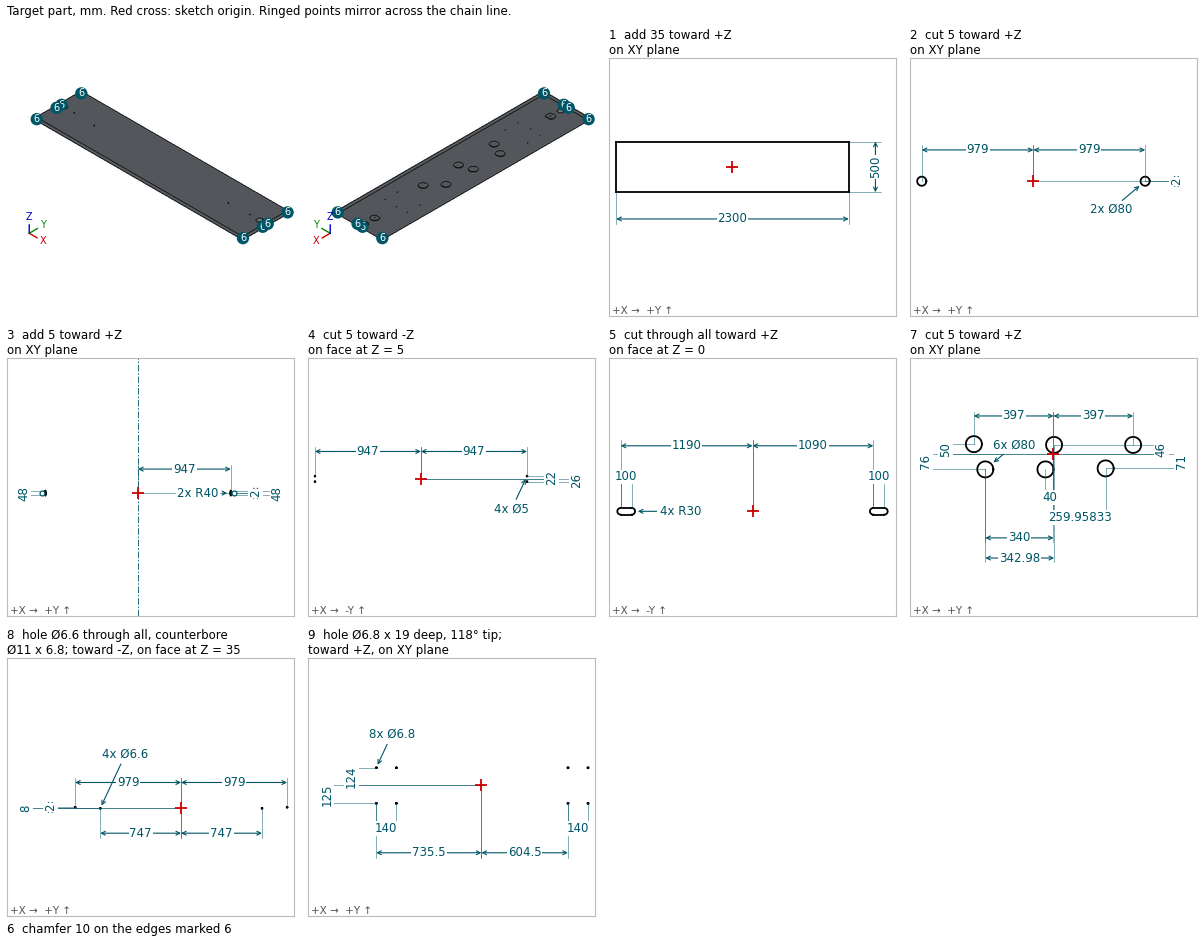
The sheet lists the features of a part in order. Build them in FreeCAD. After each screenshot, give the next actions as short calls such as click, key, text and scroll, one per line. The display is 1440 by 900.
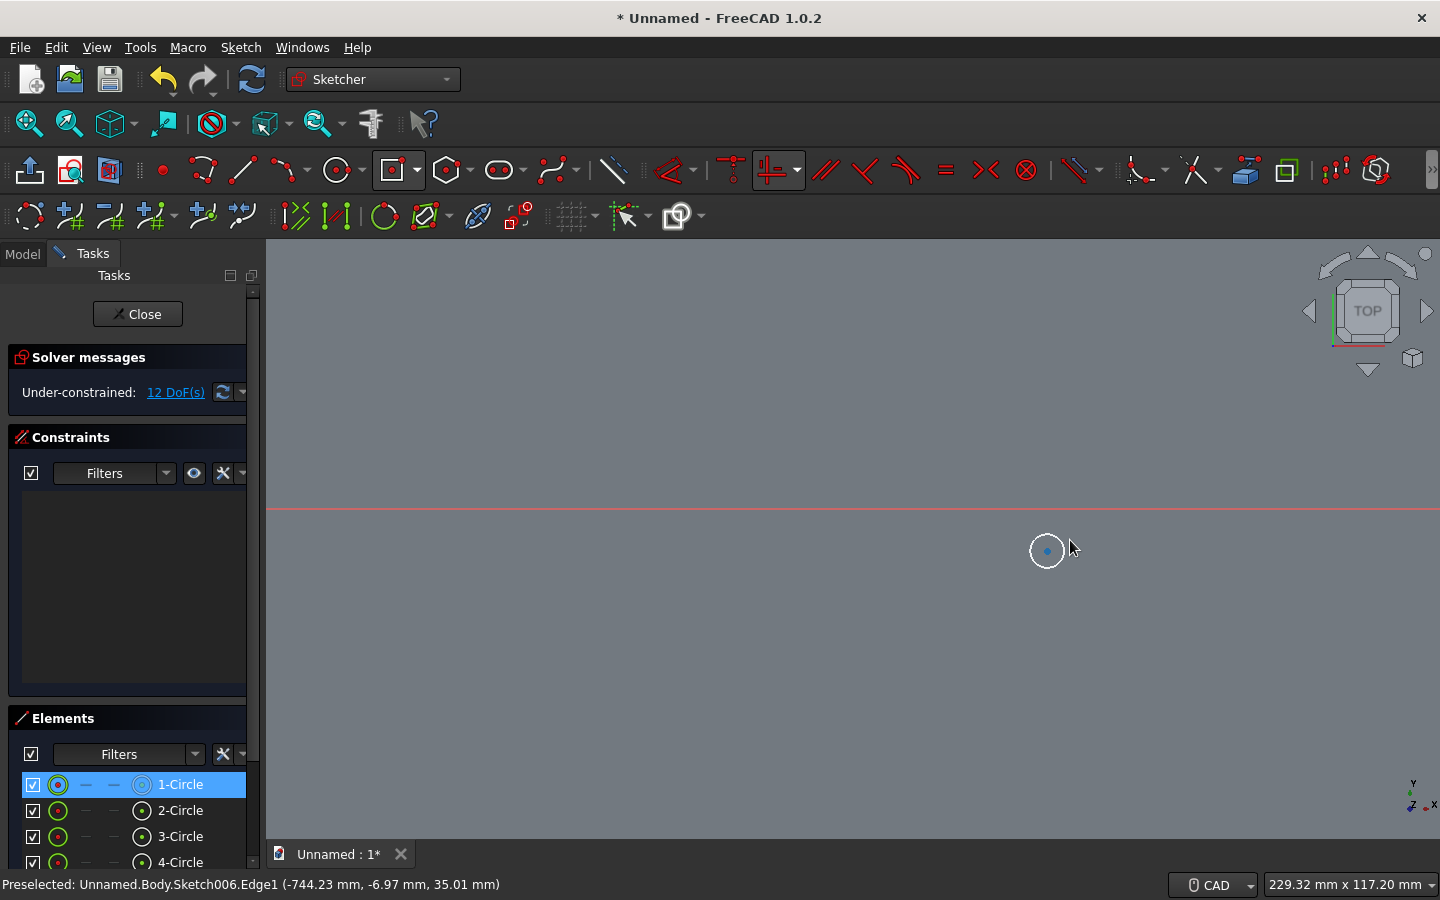
click(1059, 539)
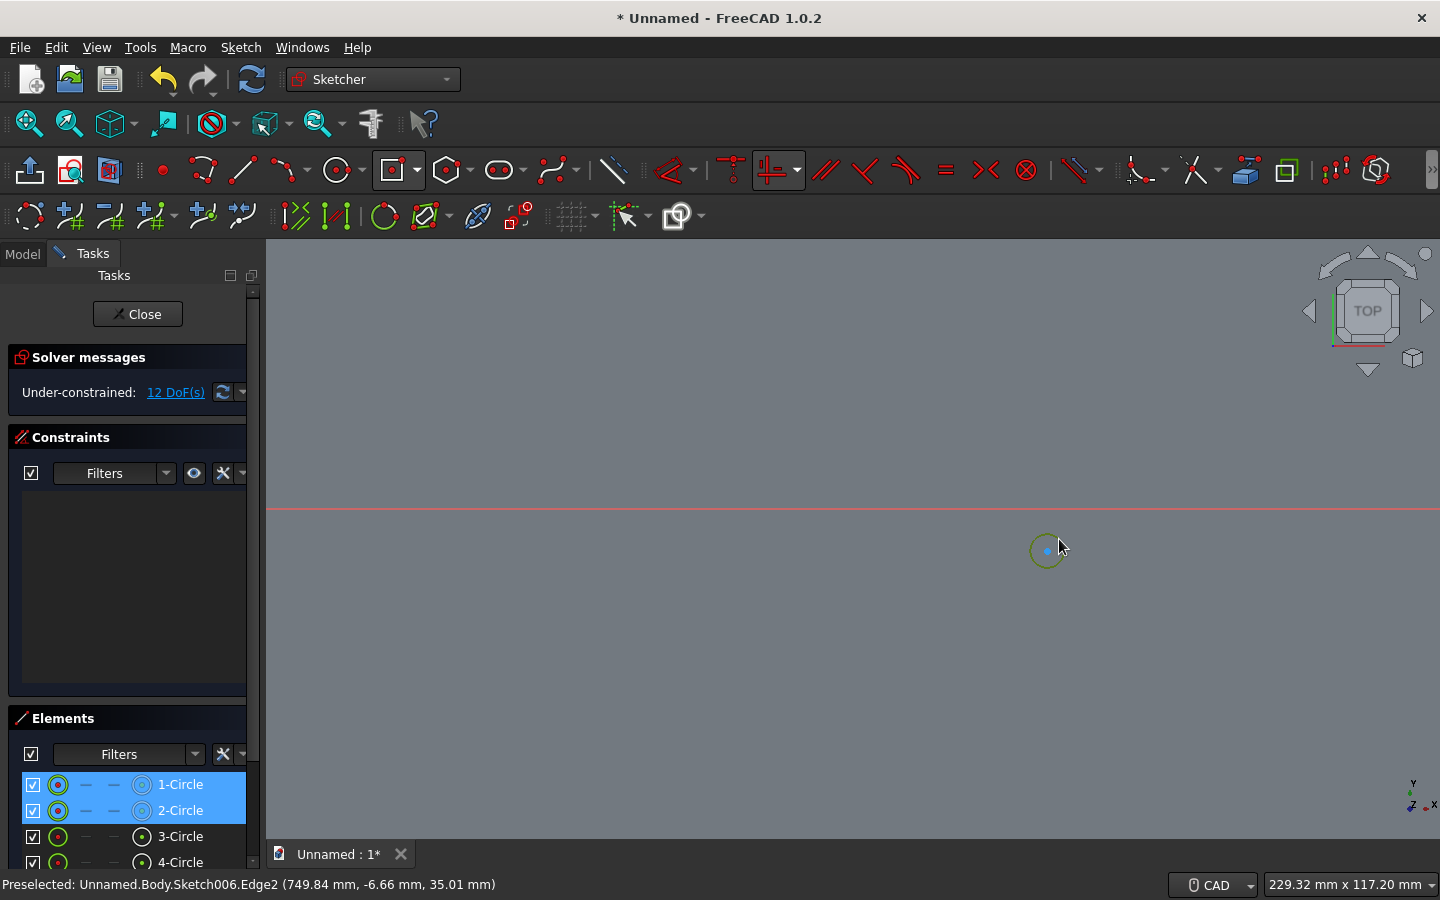
scroll(1070, 540, down, 13)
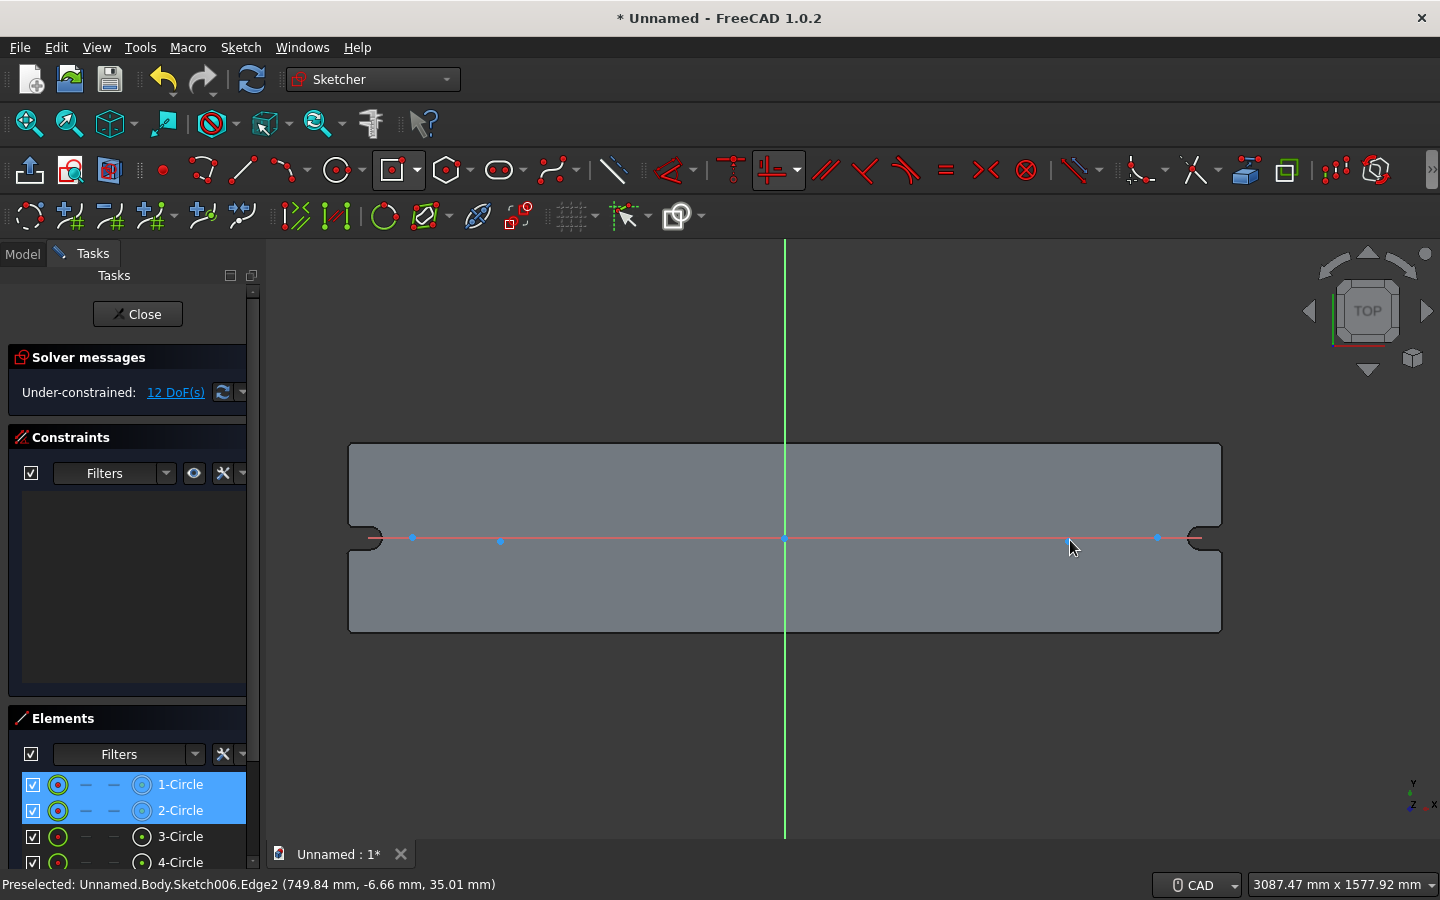
scroll(414, 537, up, 12)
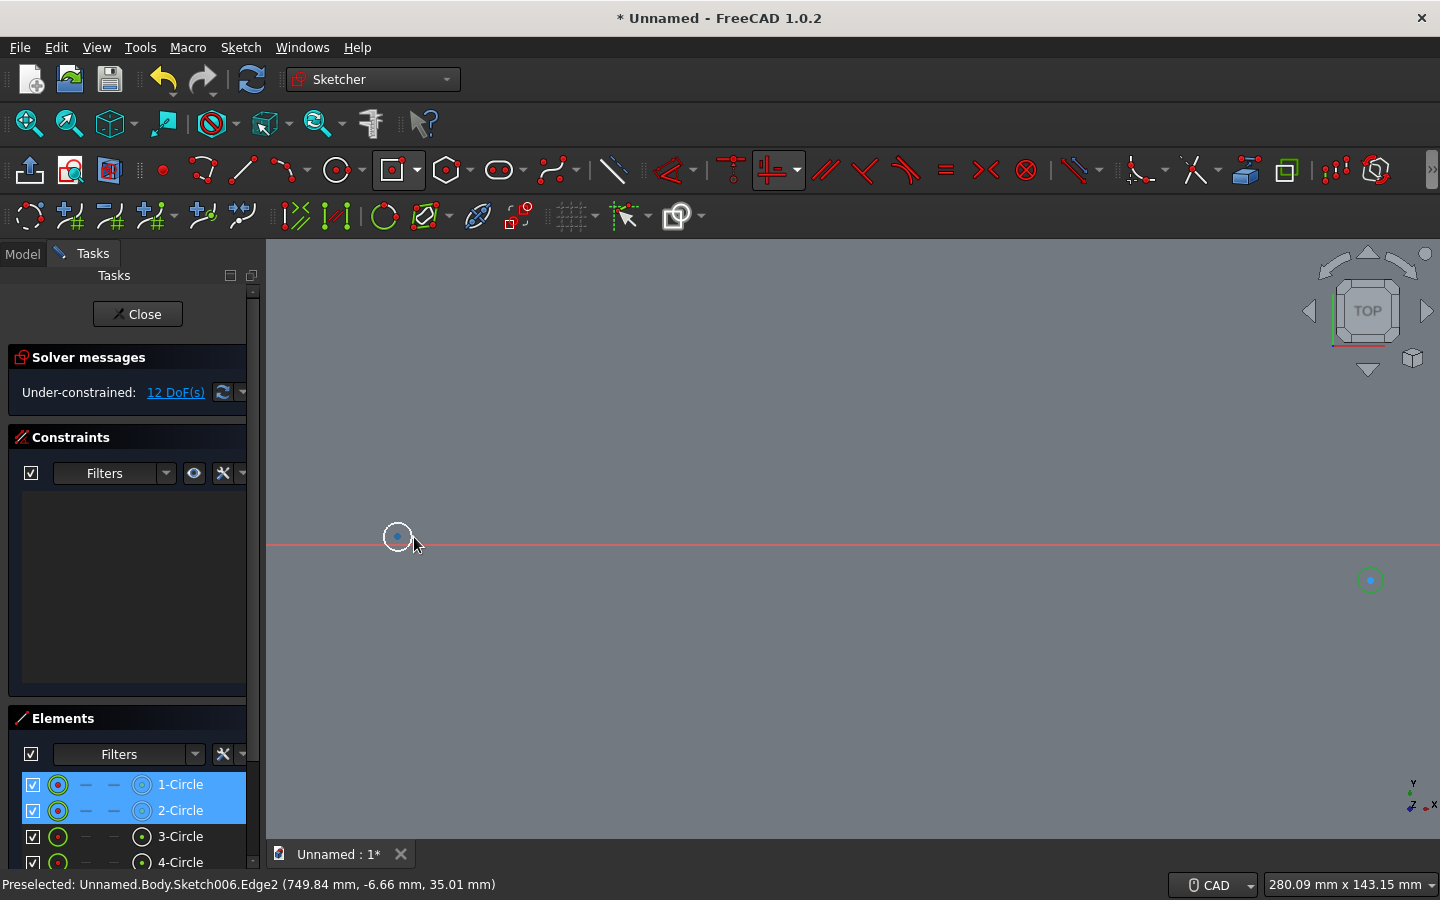
click(408, 527)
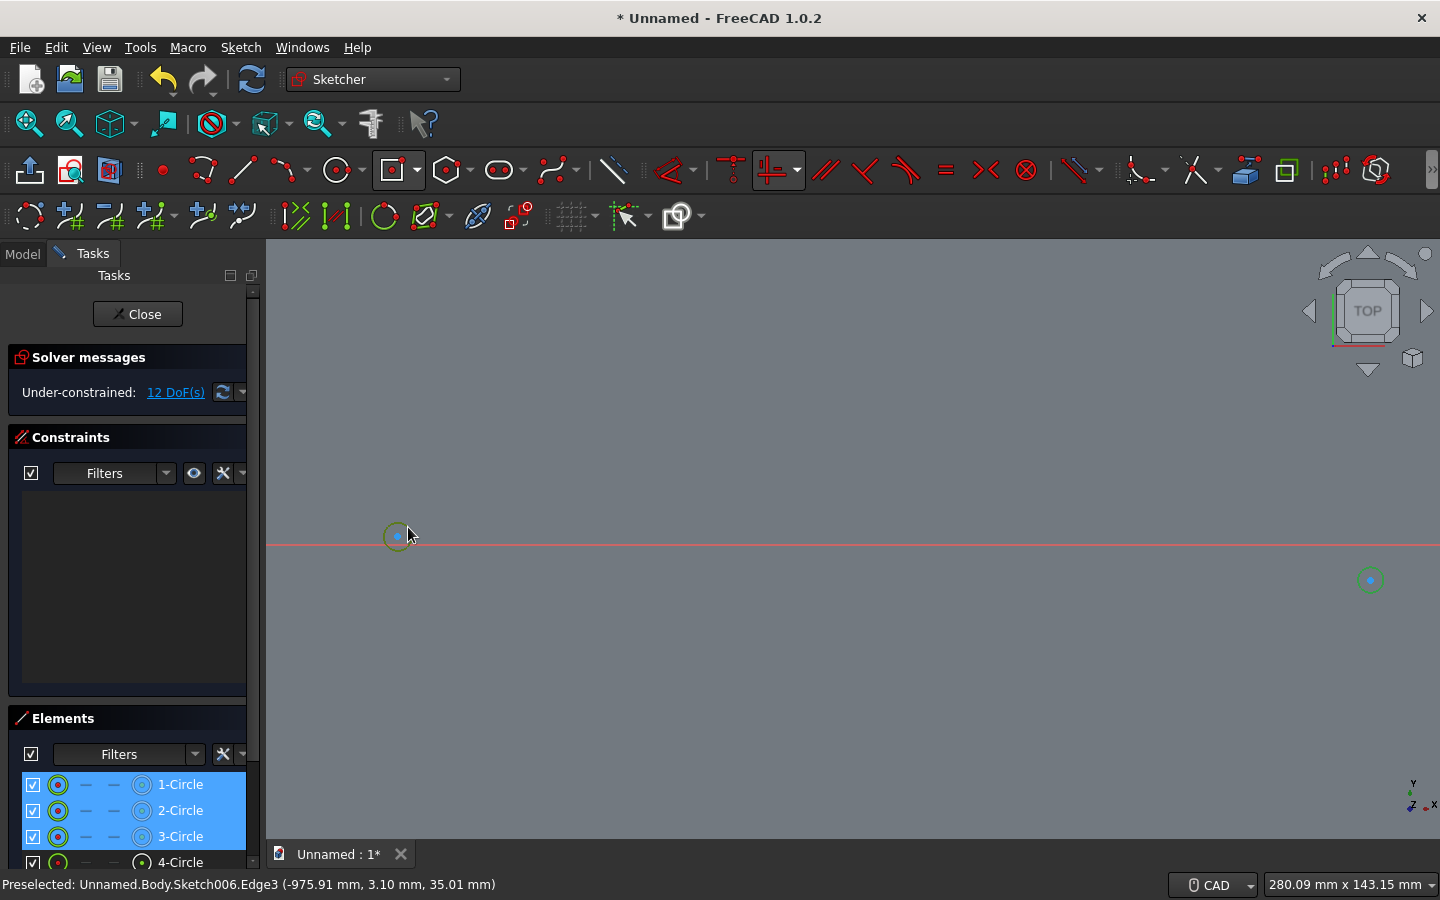
scroll(414, 537, down, 12)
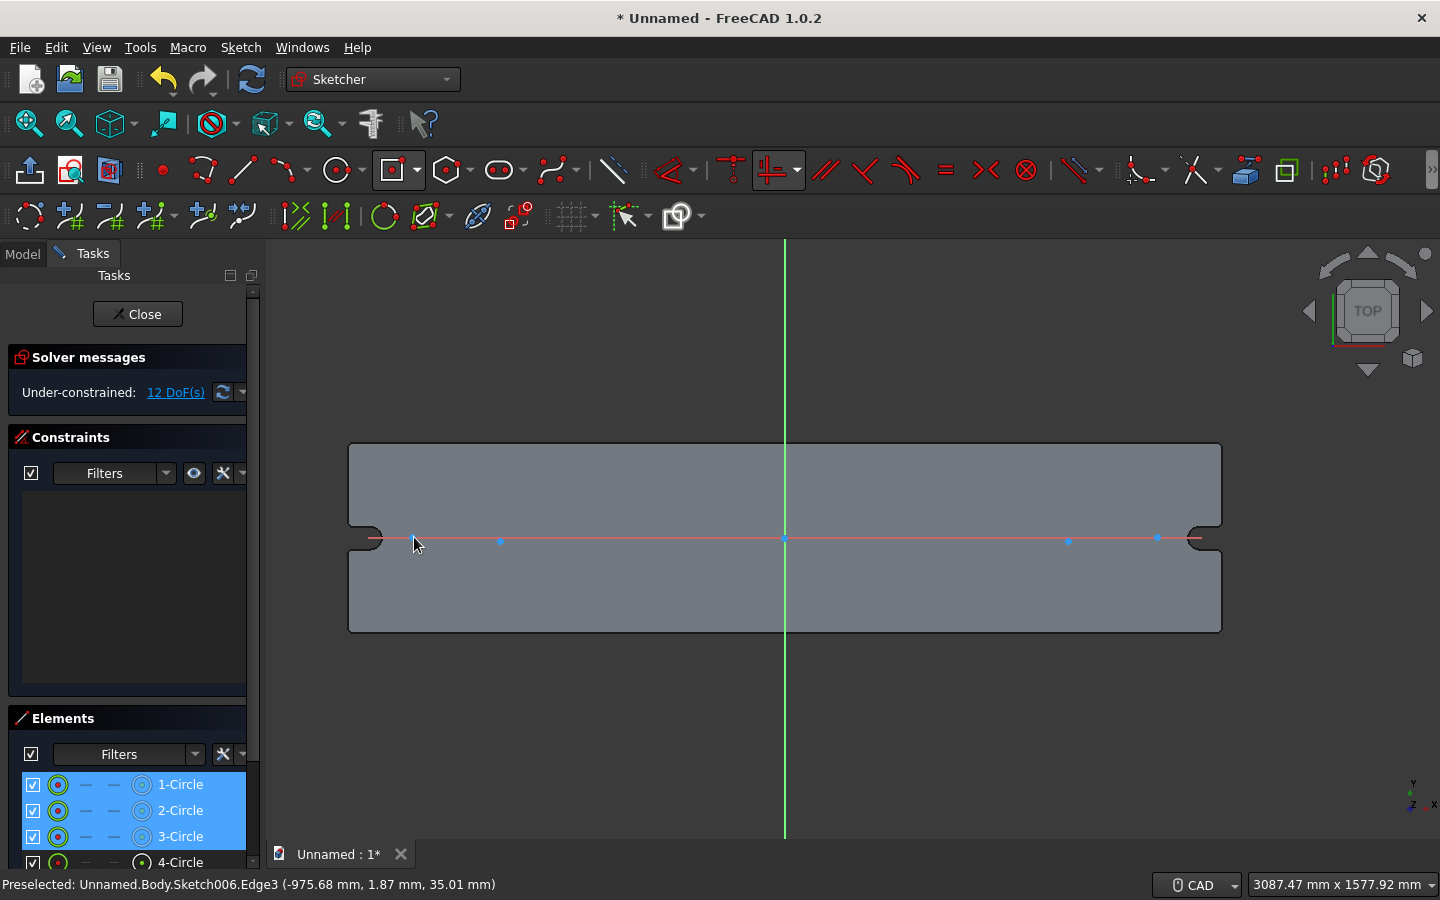
scroll(1158, 537, up, 12)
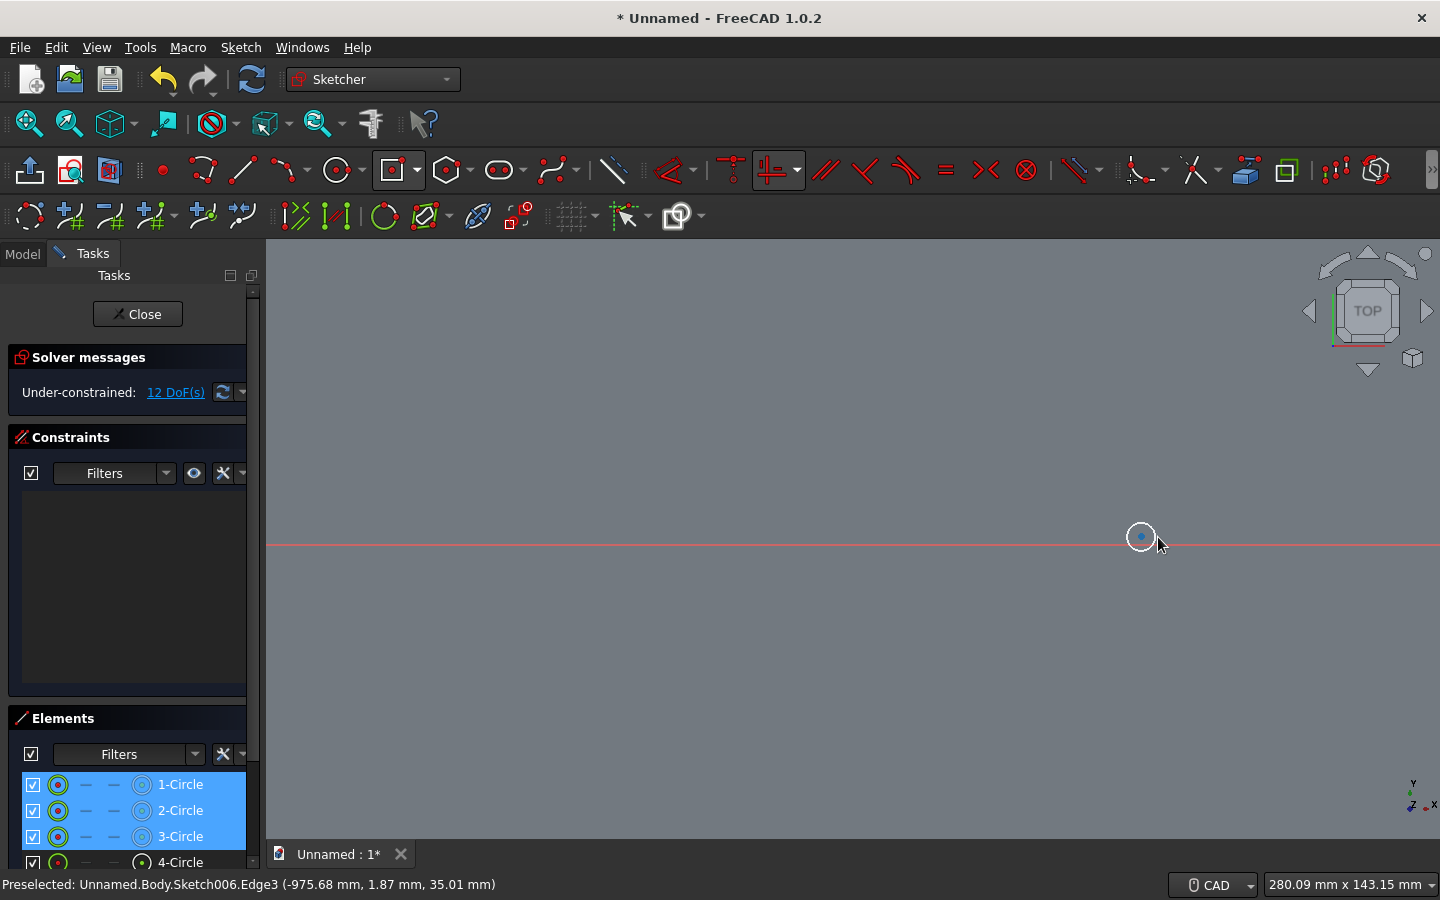
click(1151, 527)